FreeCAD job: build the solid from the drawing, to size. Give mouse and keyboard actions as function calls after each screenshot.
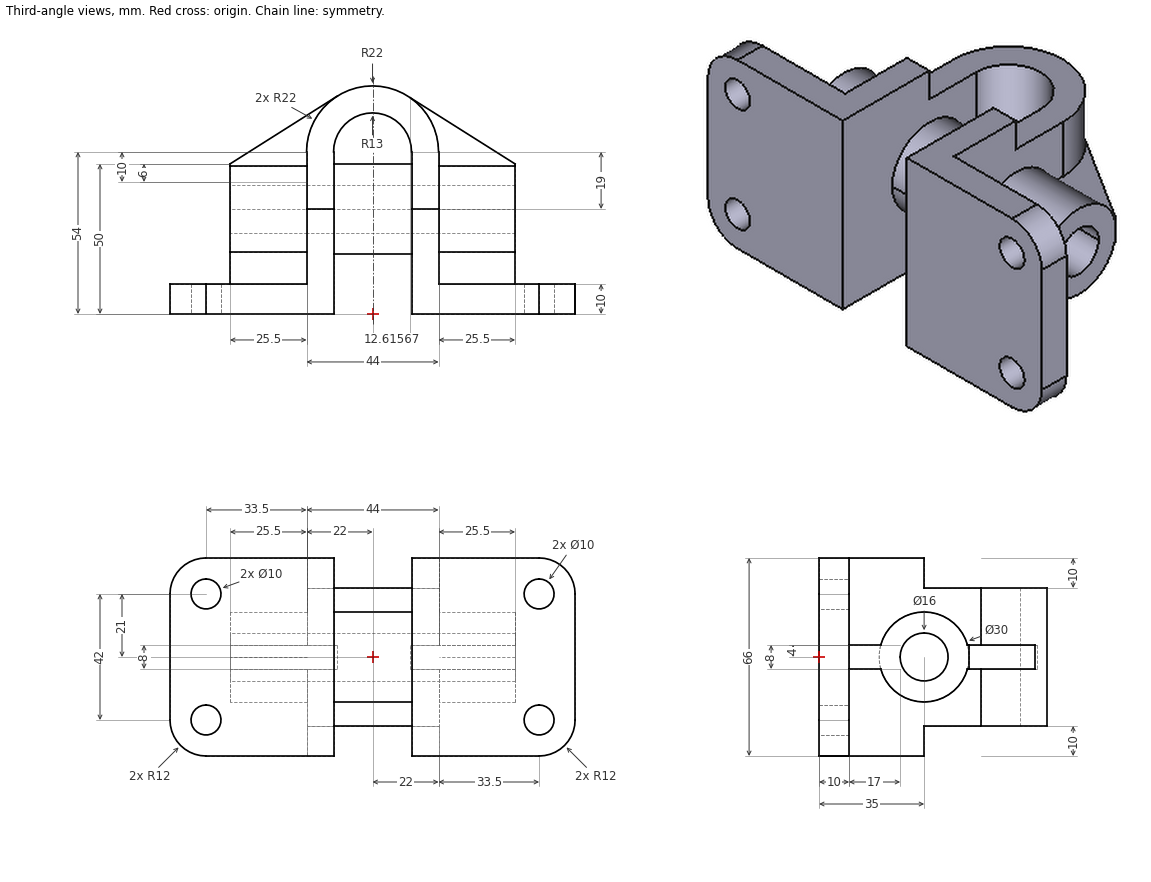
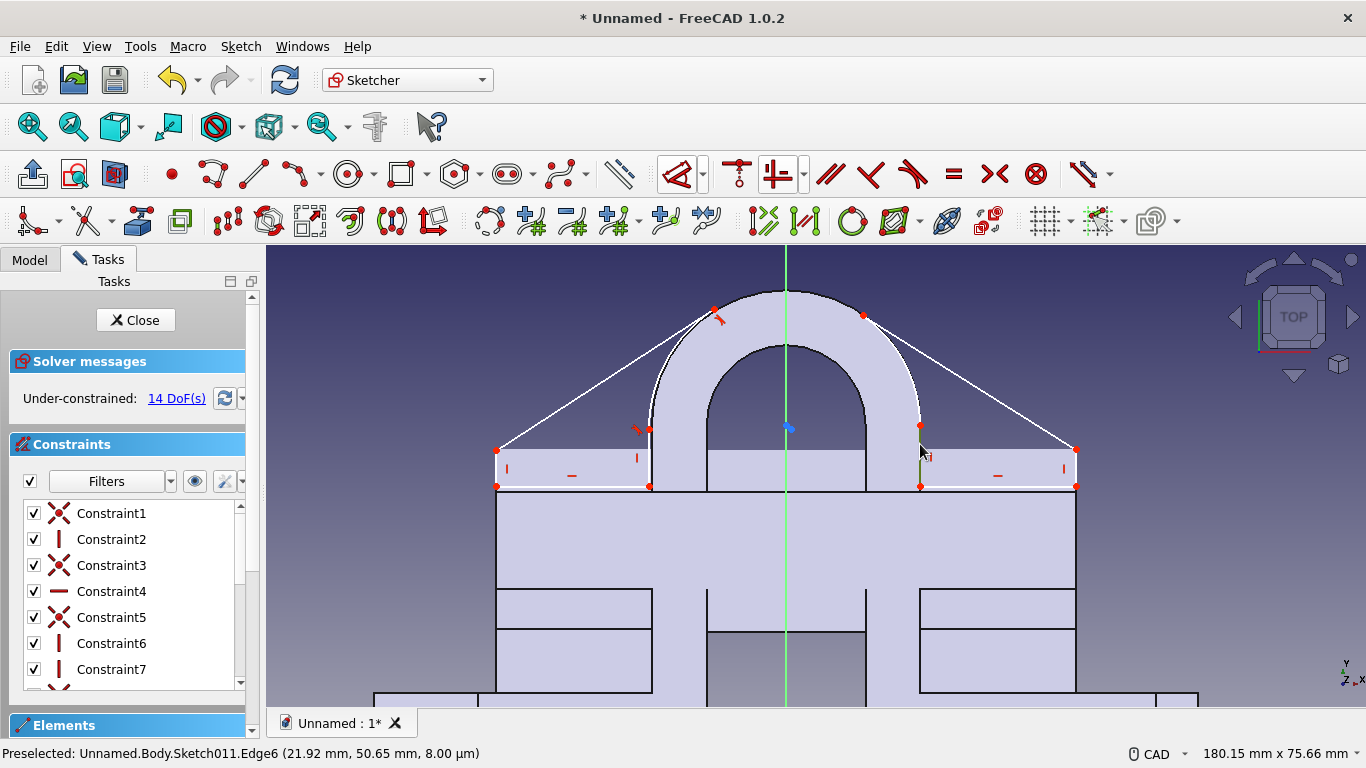
click(915, 388)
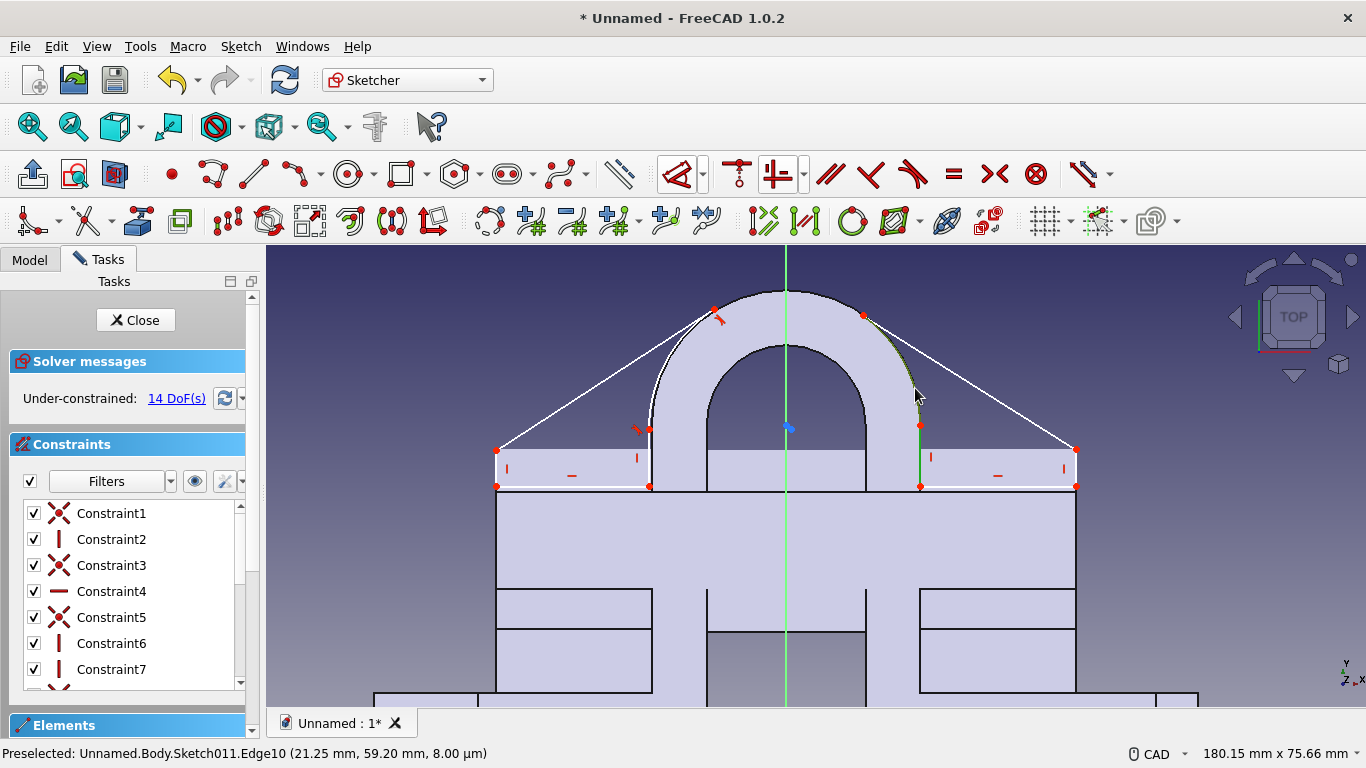
click(913, 174)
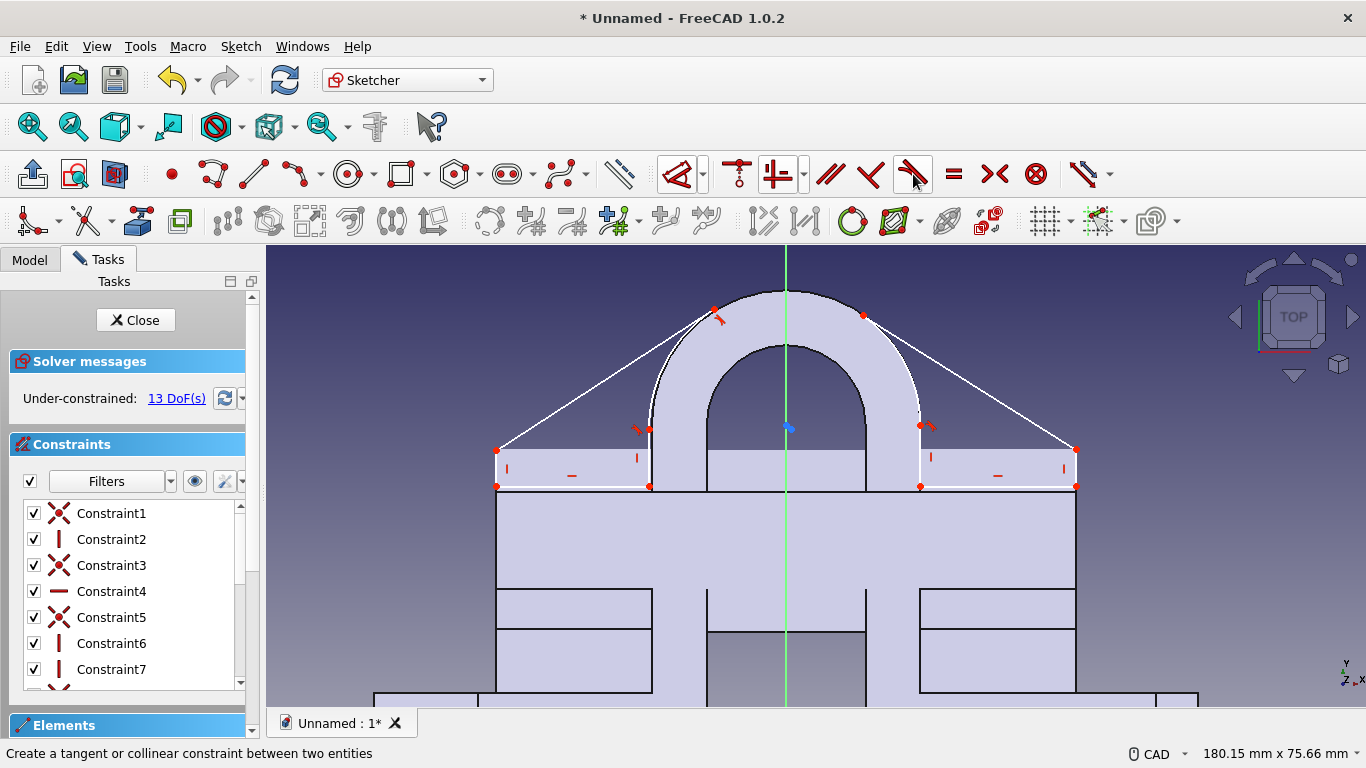
click(655, 387)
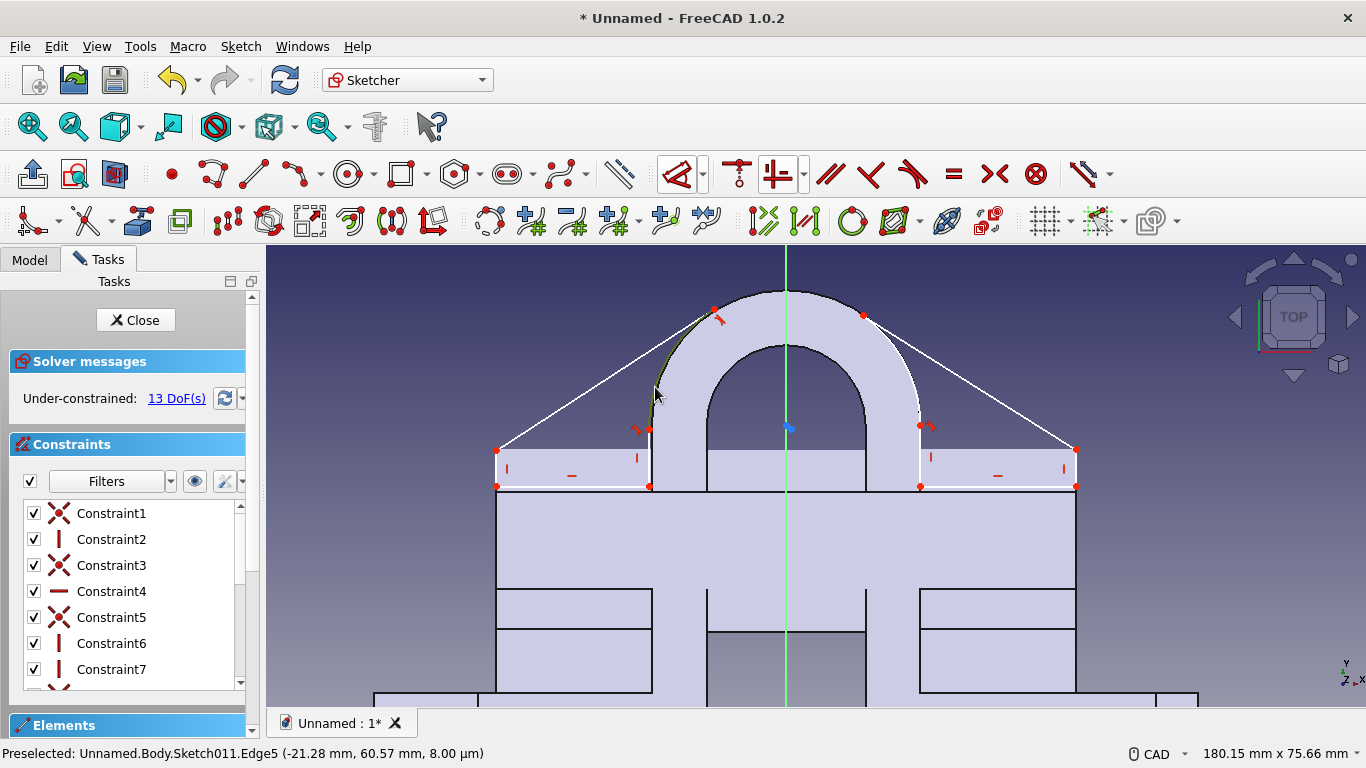
click(915, 388)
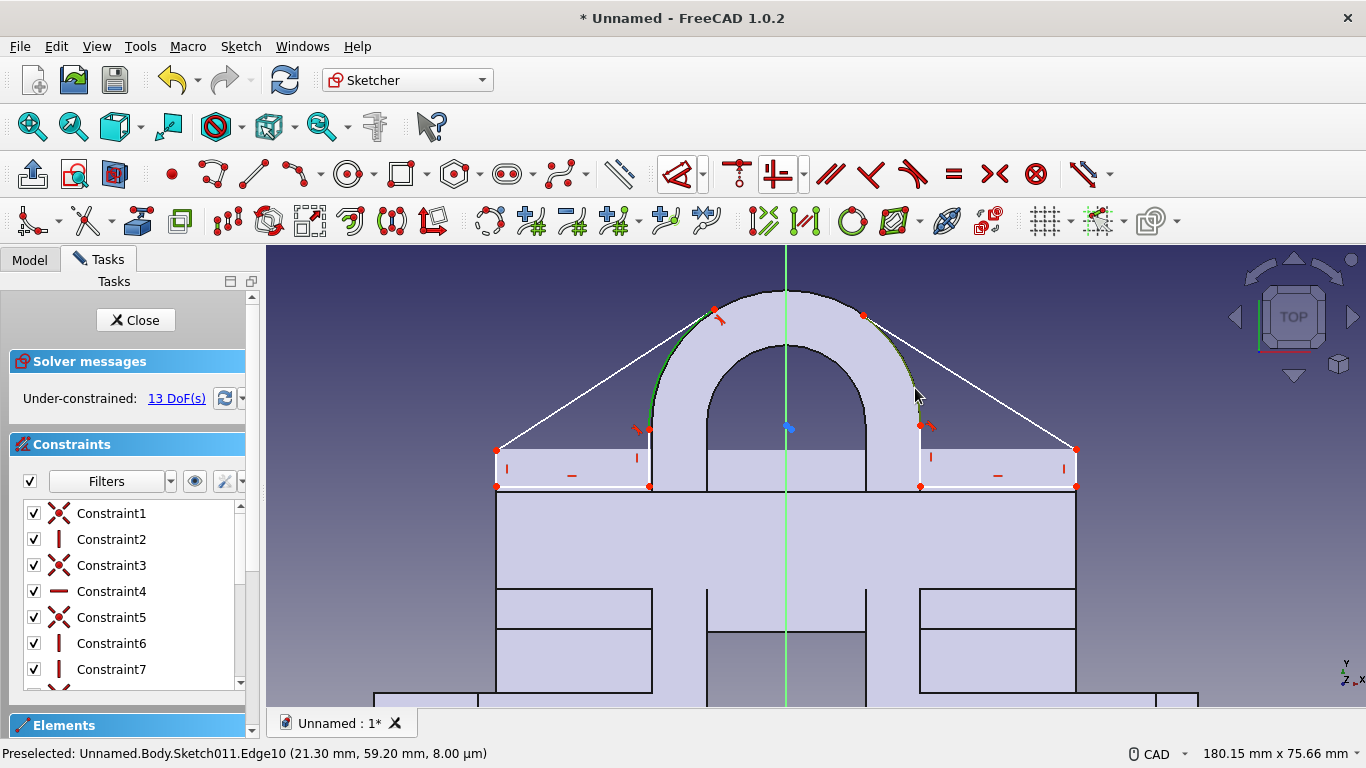
click(737, 174)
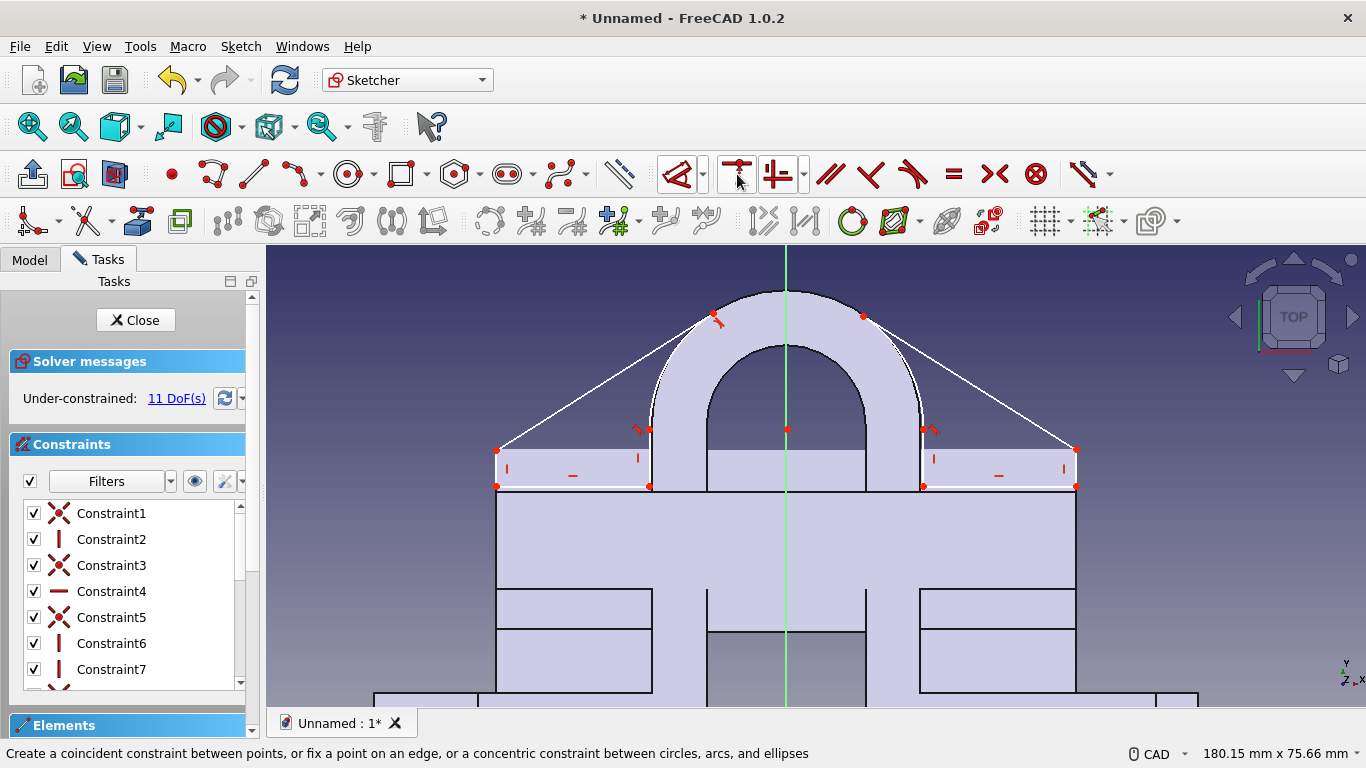
click(656, 388)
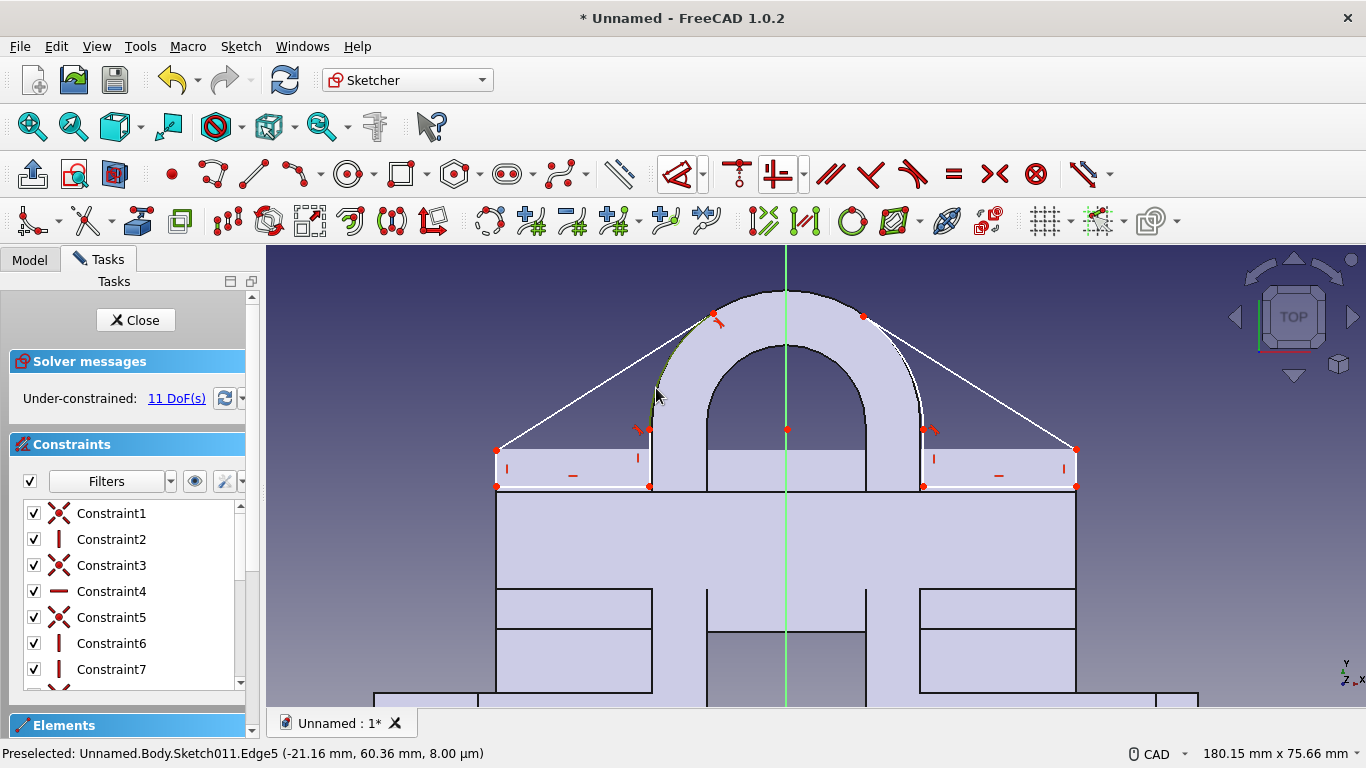
click(918, 390)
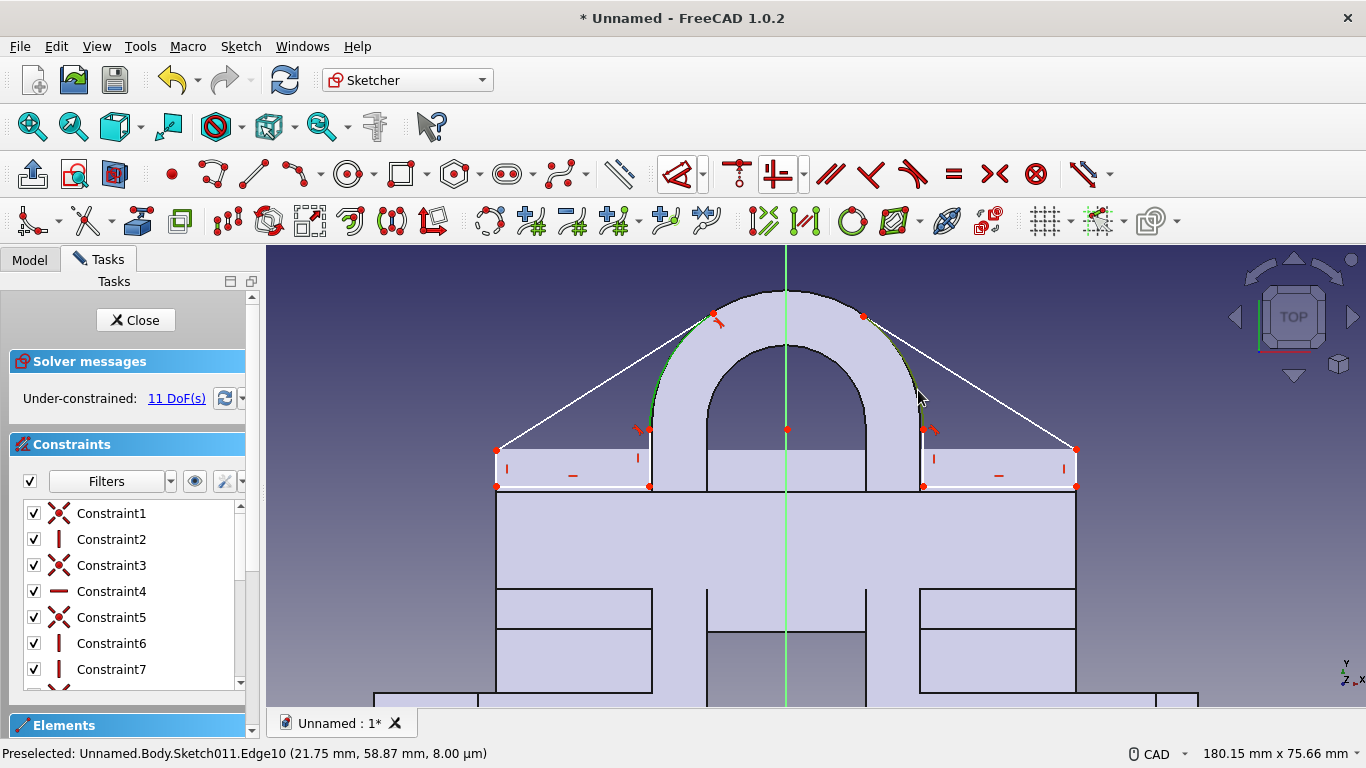
click(954, 174)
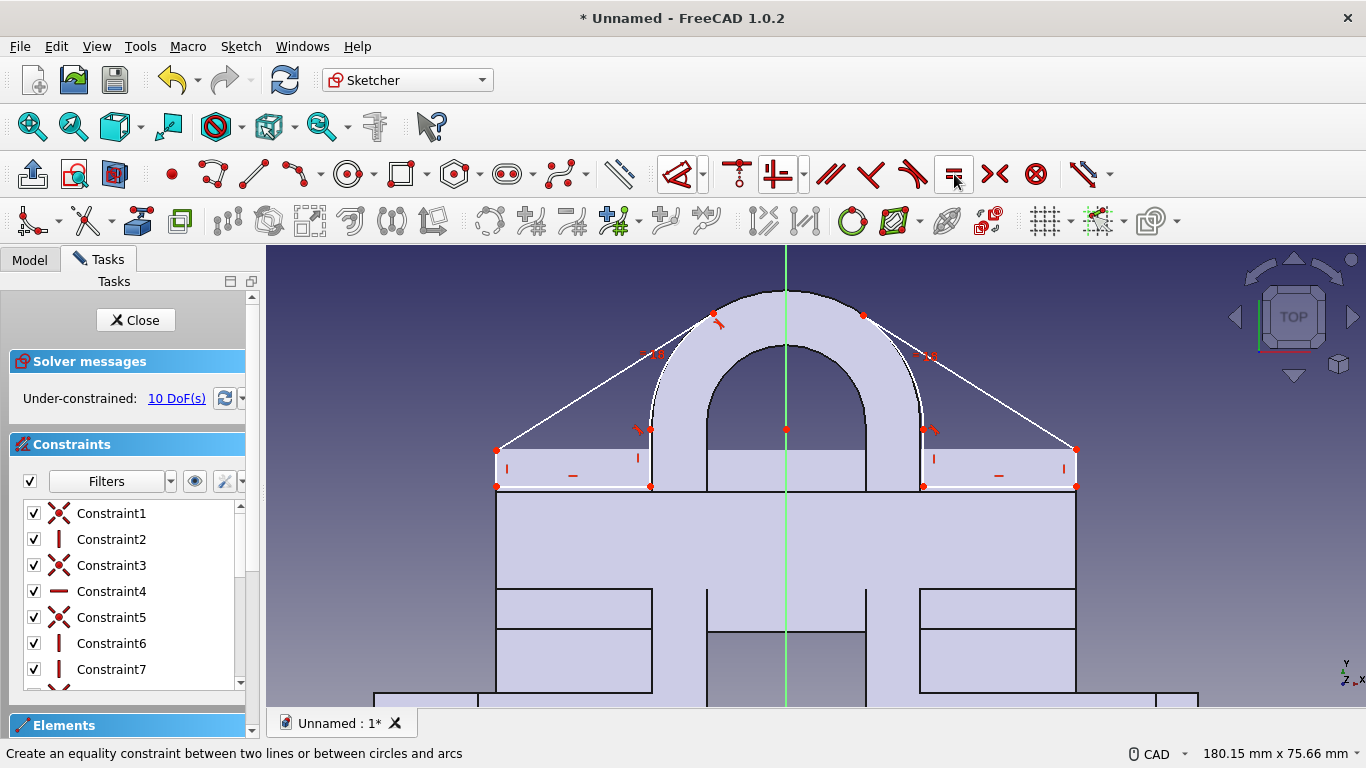
click(787, 429)